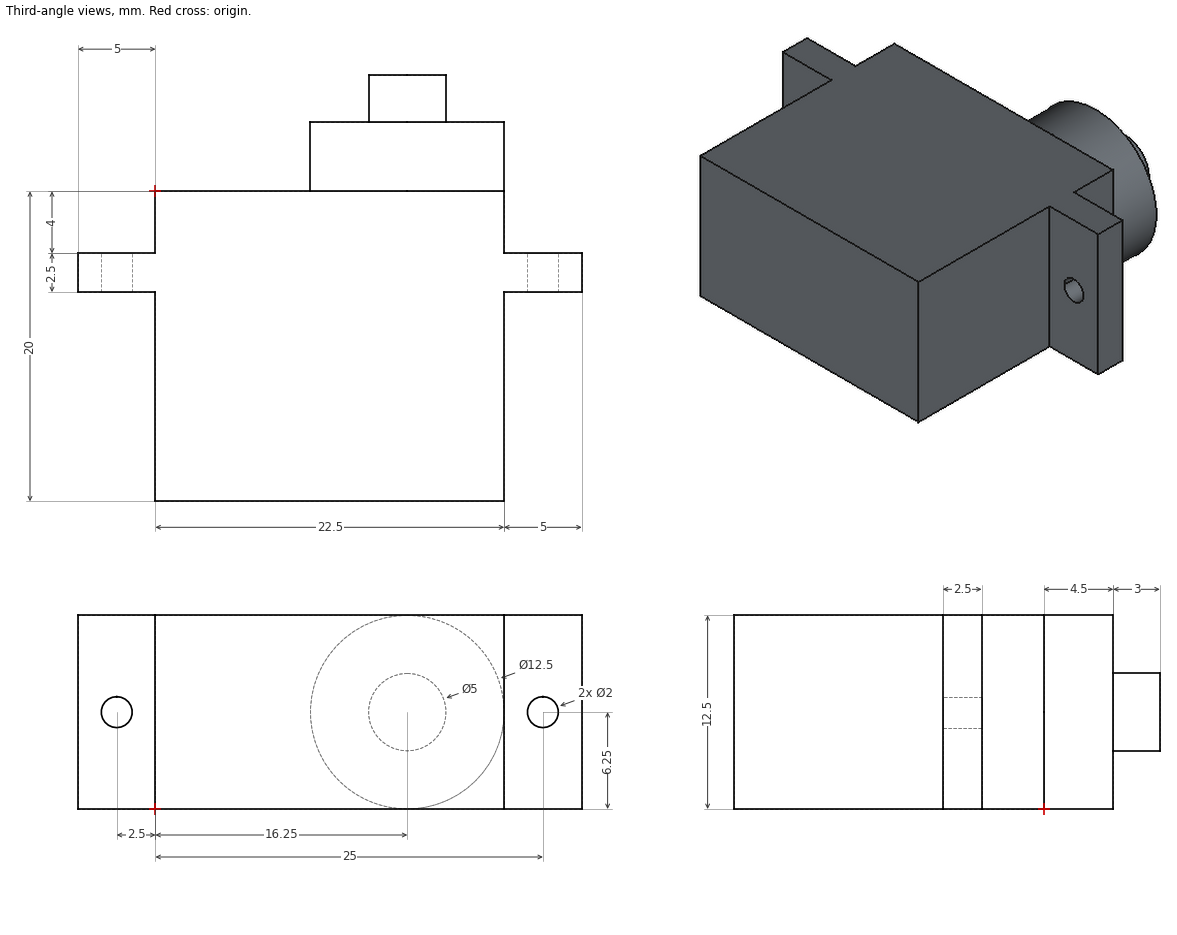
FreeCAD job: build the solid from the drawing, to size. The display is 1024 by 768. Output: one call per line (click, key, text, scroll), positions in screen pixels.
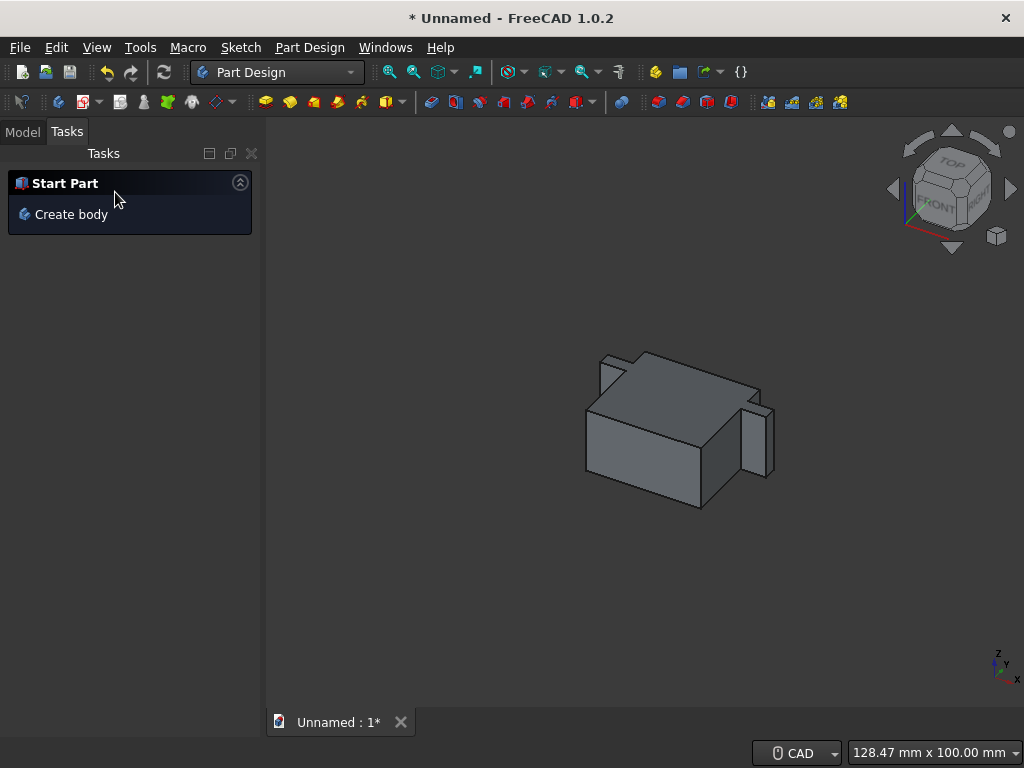
key(v)
key(f)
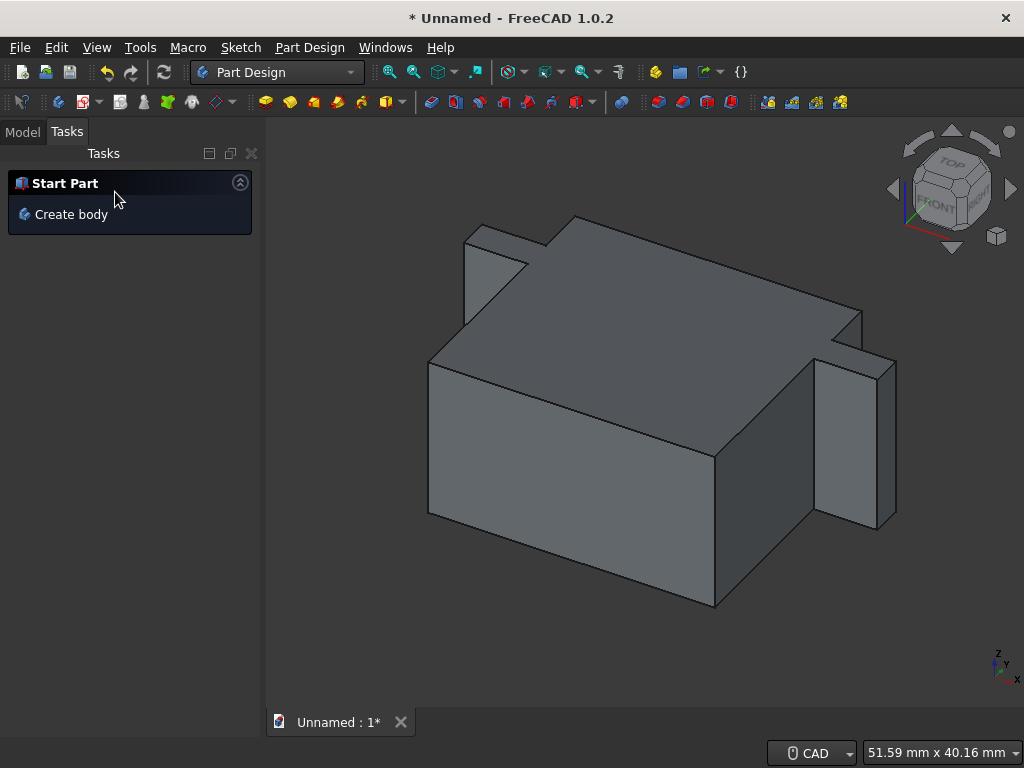
key(4)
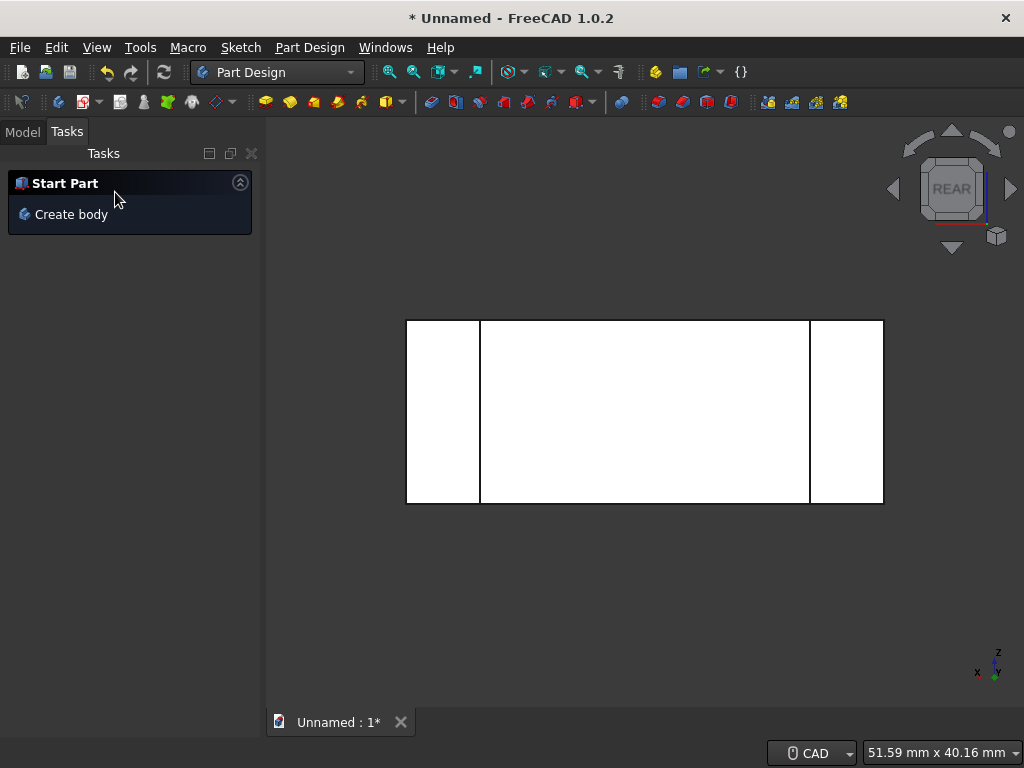
click(847, 359)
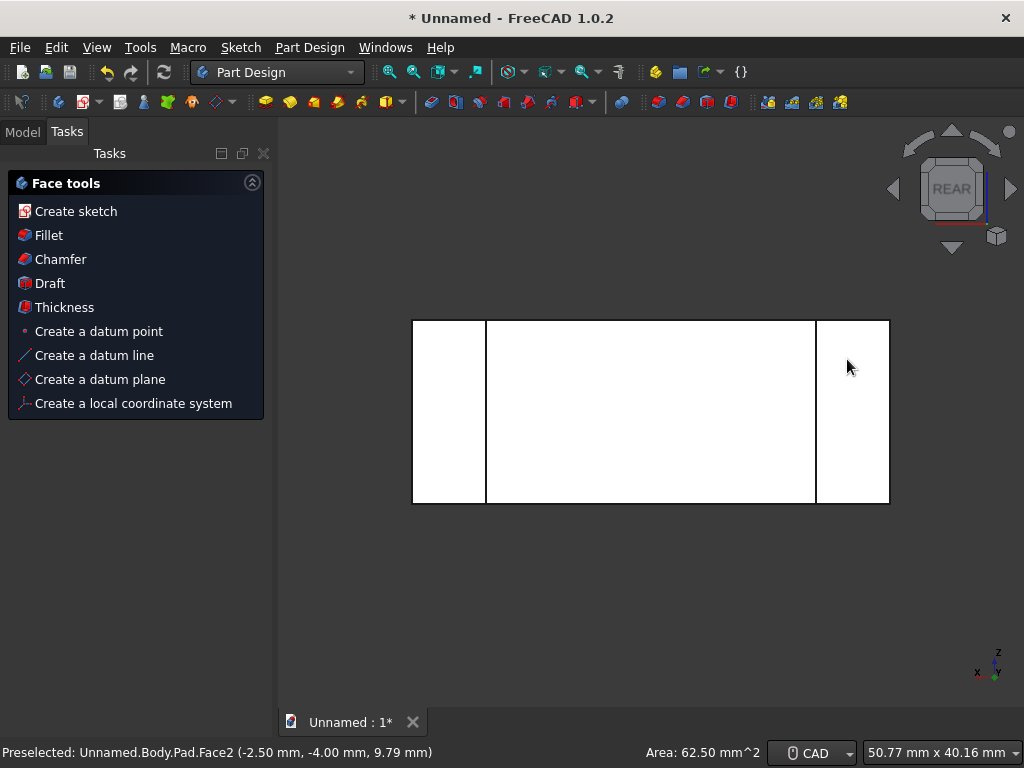
click(84, 102)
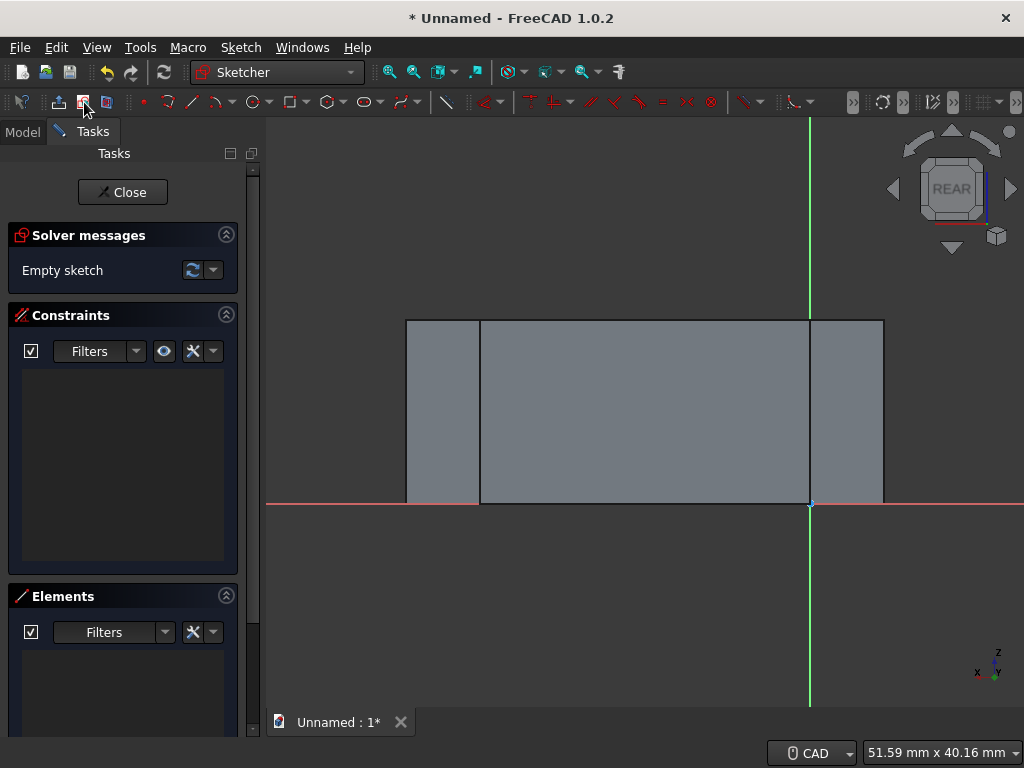
scroll(294, 238, down, 1)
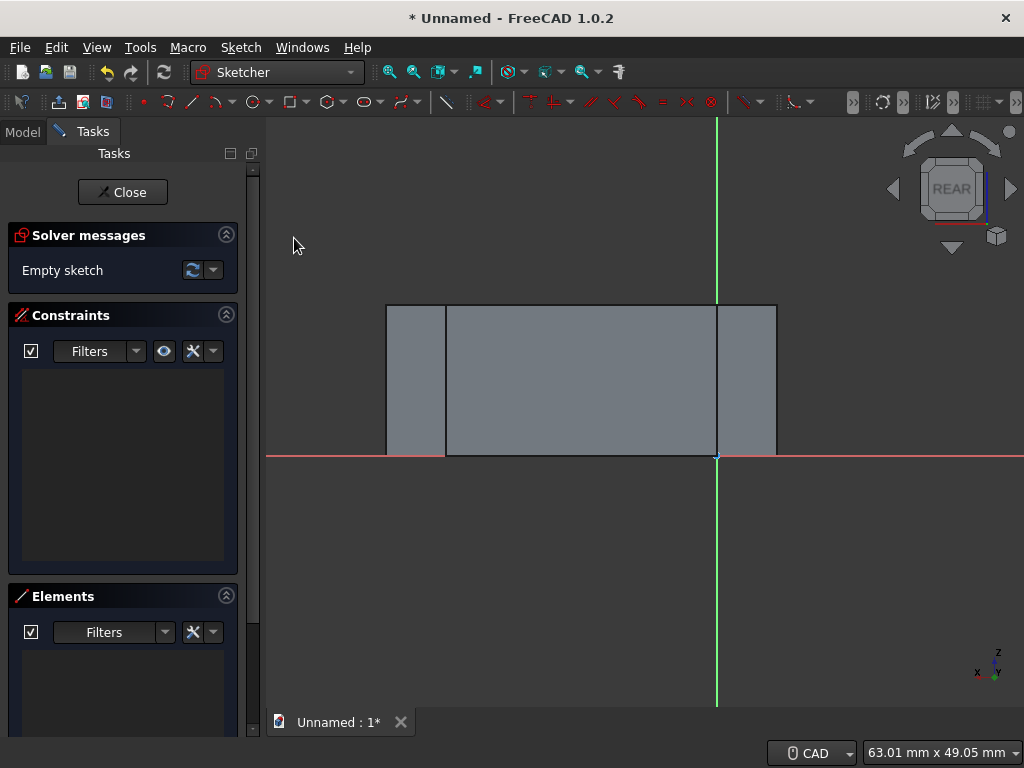
key(g)
key(c)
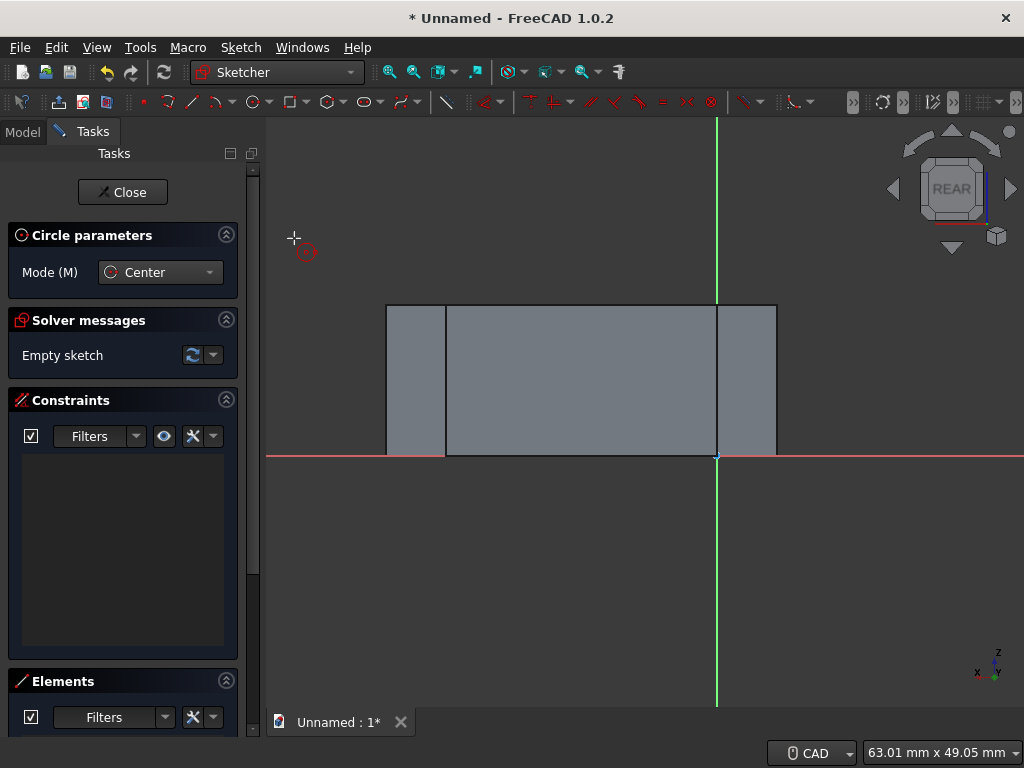
scroll(416, 380, up, 4)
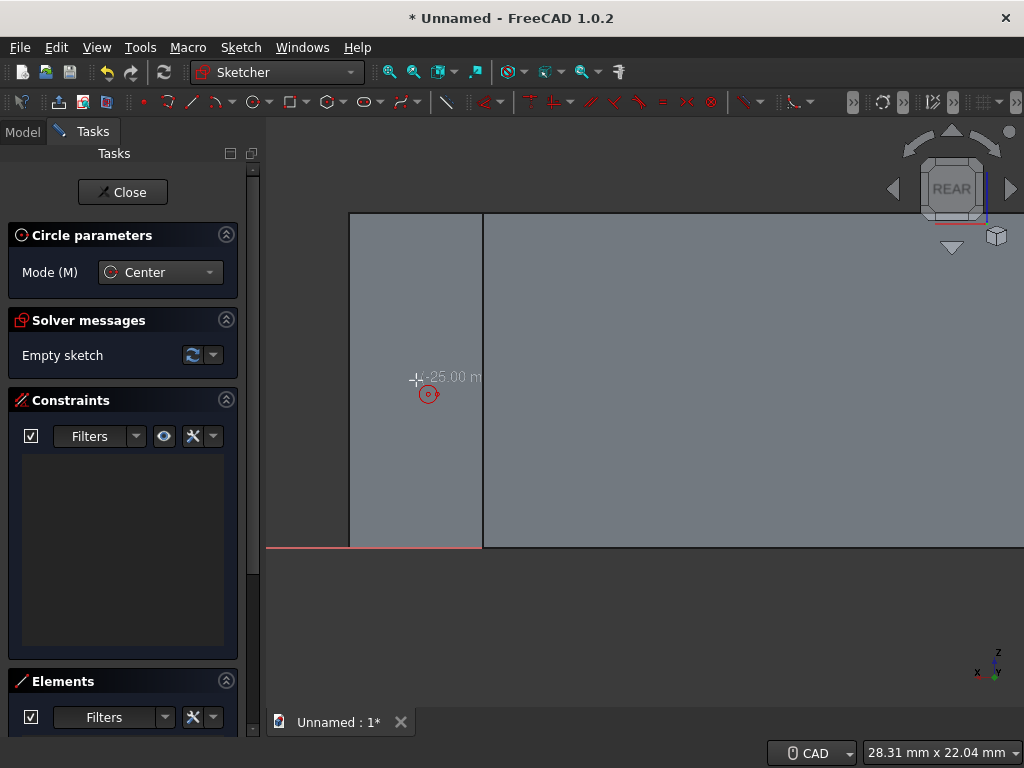
click(416, 381)
move(435, 362)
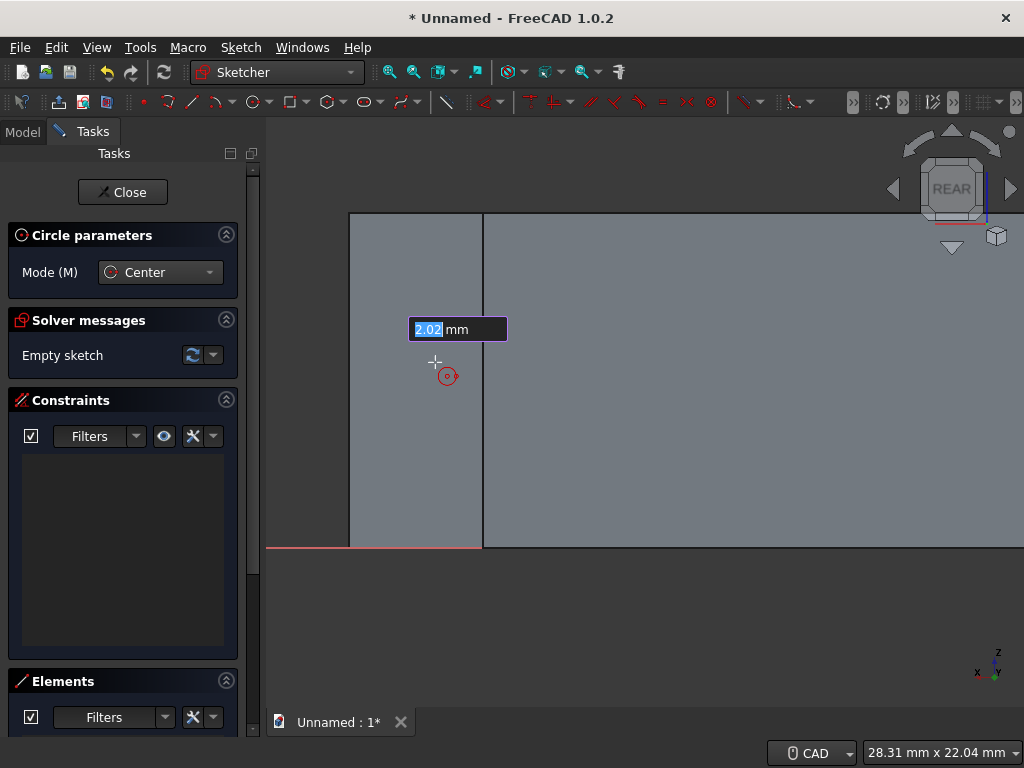
text(2)
key(Return)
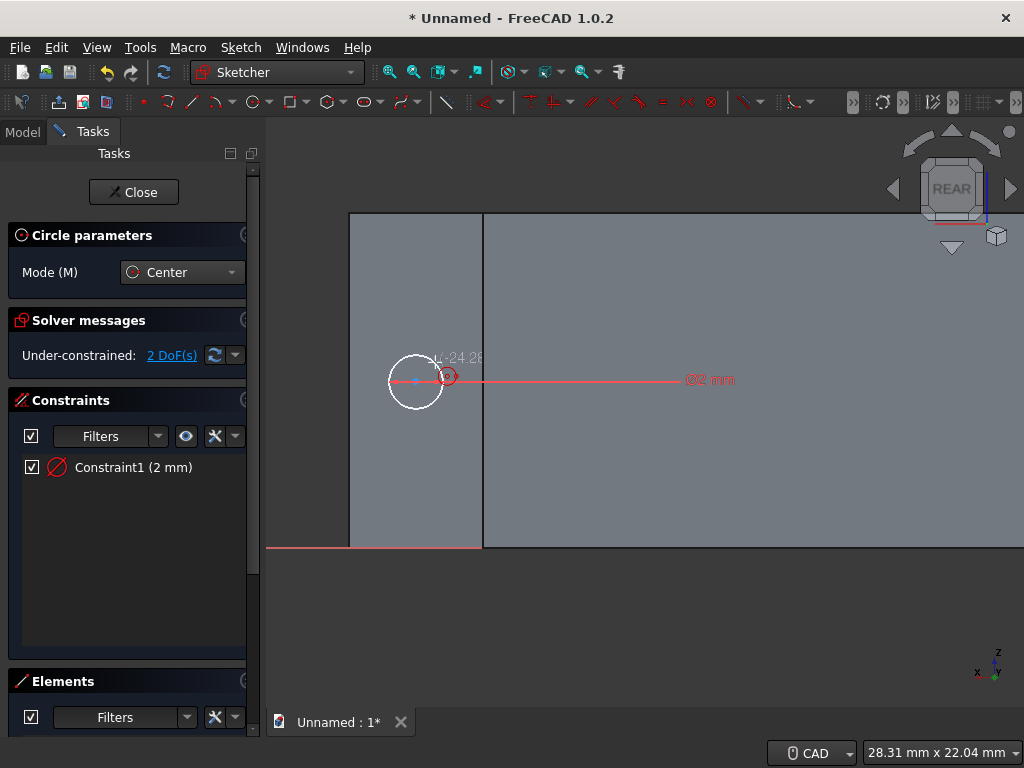
scroll(324, 365, down, 3)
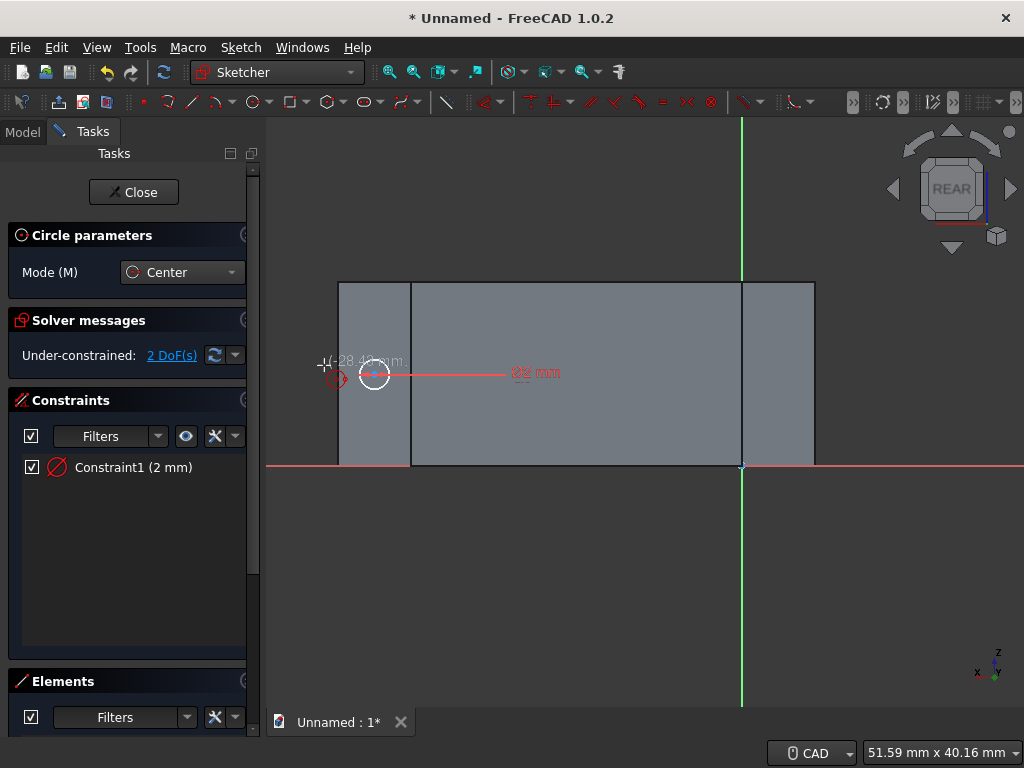
scroll(778, 374, up, 3)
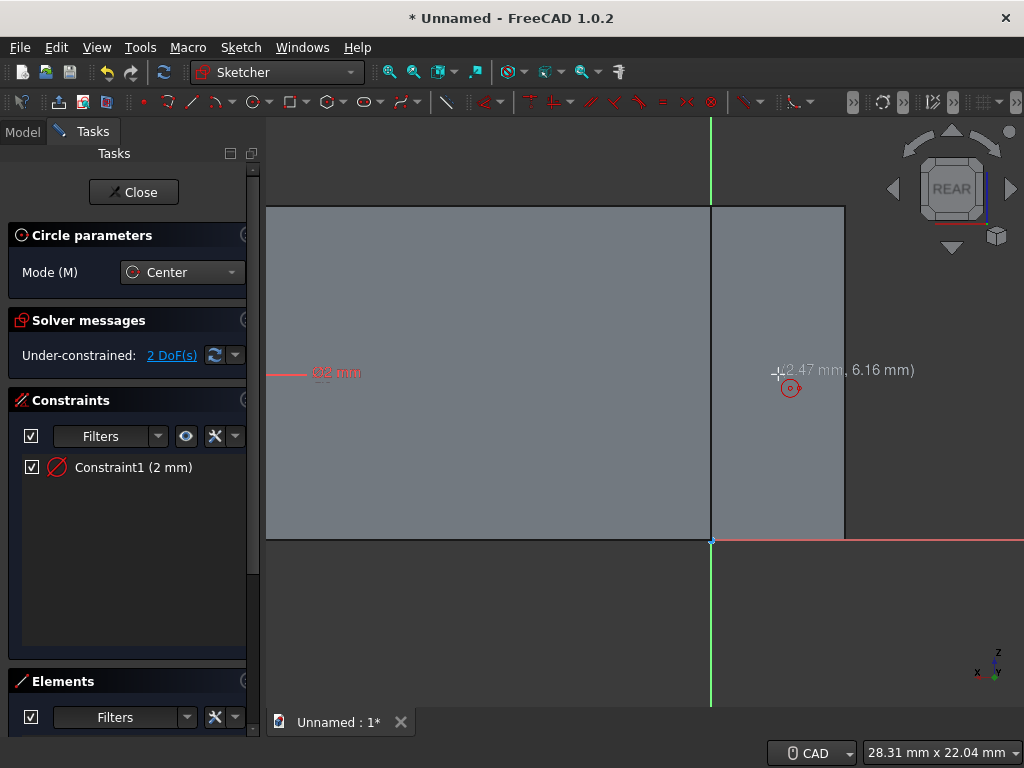
click(778, 373)
move(797, 354)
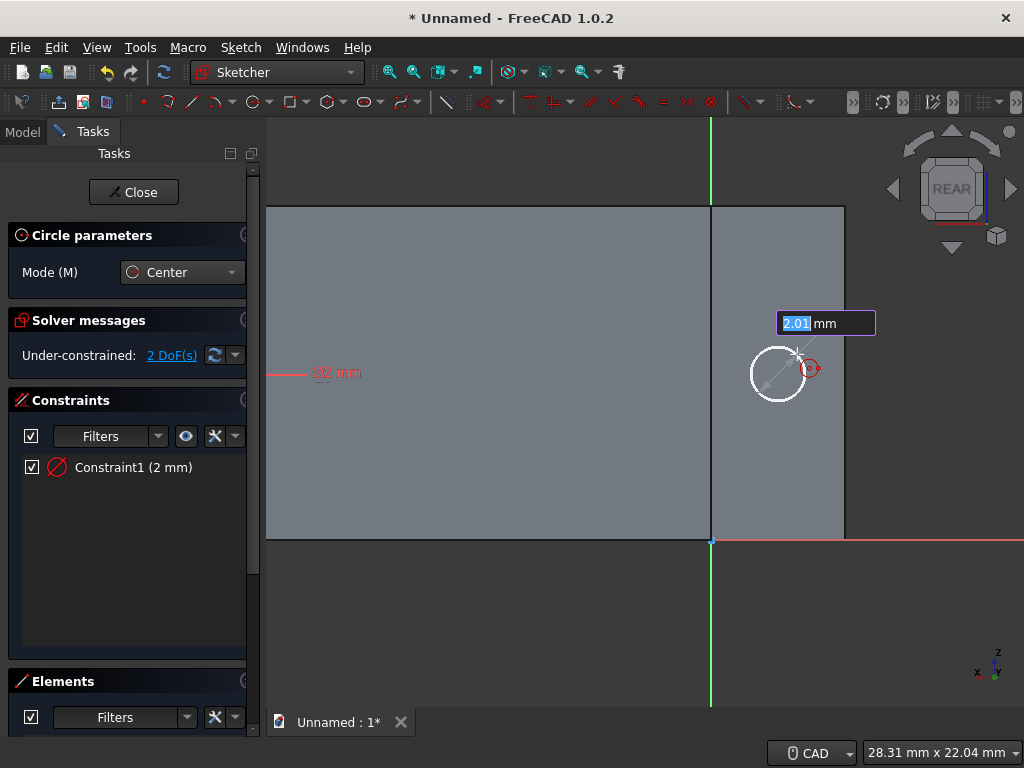
text(2)
key(Return)
key(Escape)